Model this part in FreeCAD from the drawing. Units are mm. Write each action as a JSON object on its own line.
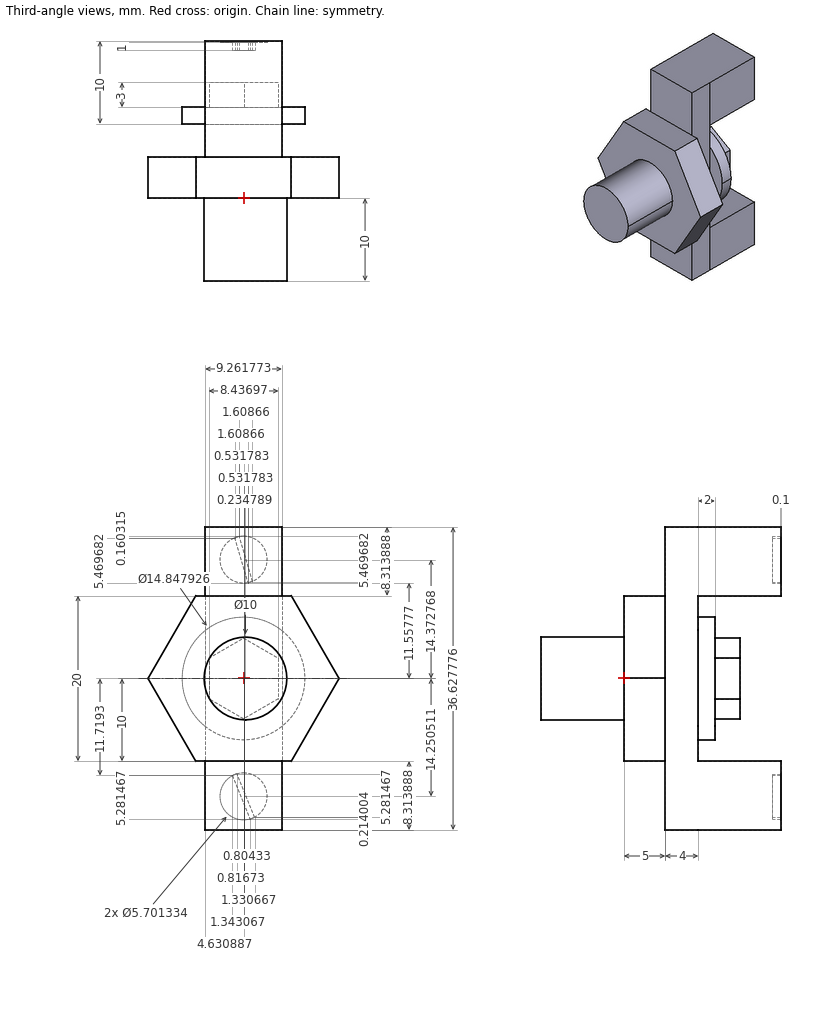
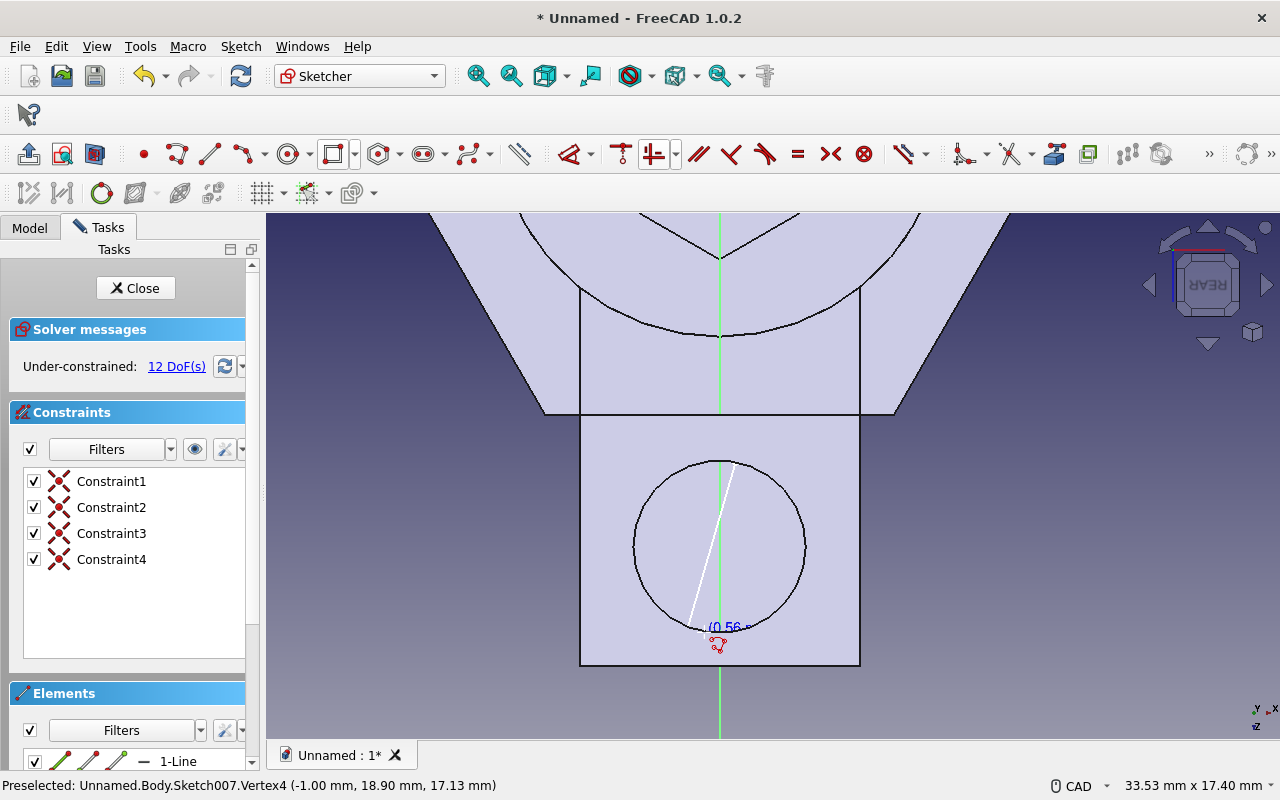
{"action": "left_click", "coordinate": [703, 632]}
{"action": "left_click", "coordinate": [752, 467]}
{"action": "left_click", "coordinate": [735, 463]}
{"action": "key", "text": "Escape"}
{"action": "key", "text": "Escape"}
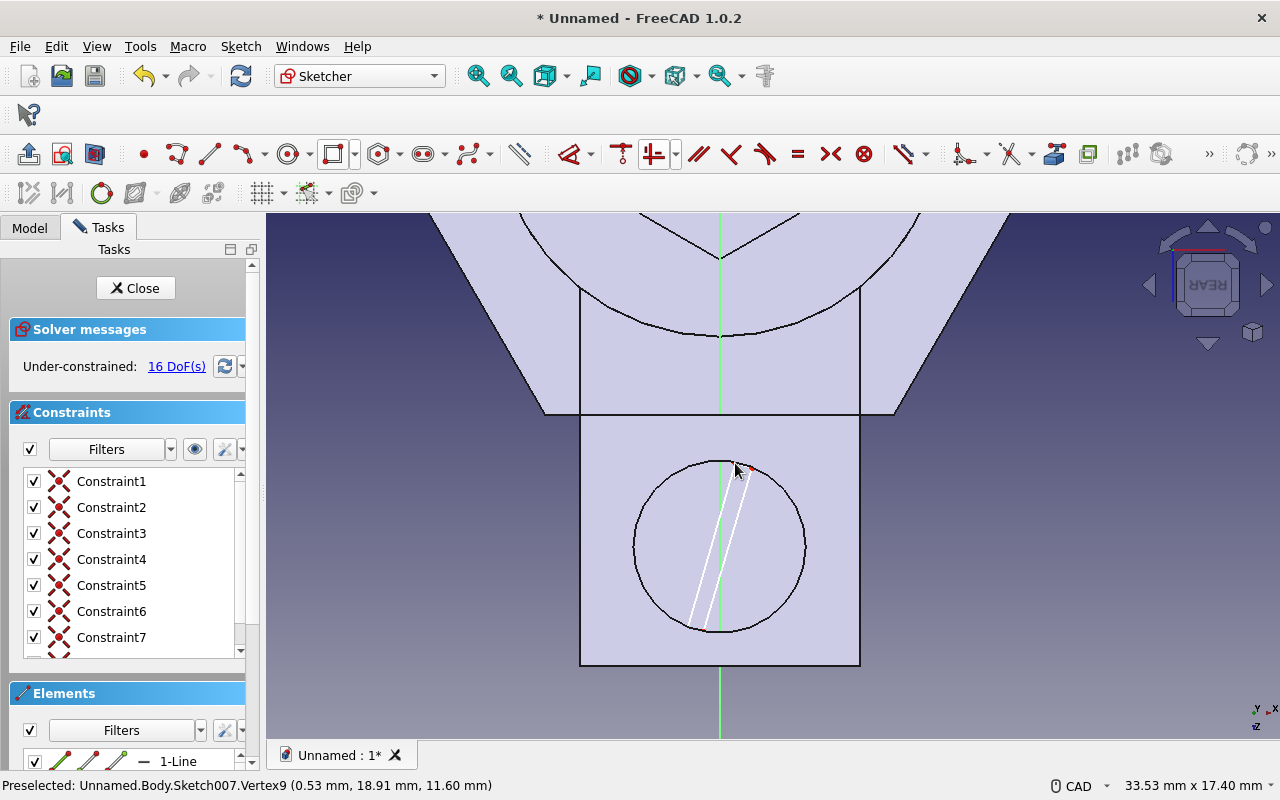
{"action": "left_click", "coordinate": [568, 154]}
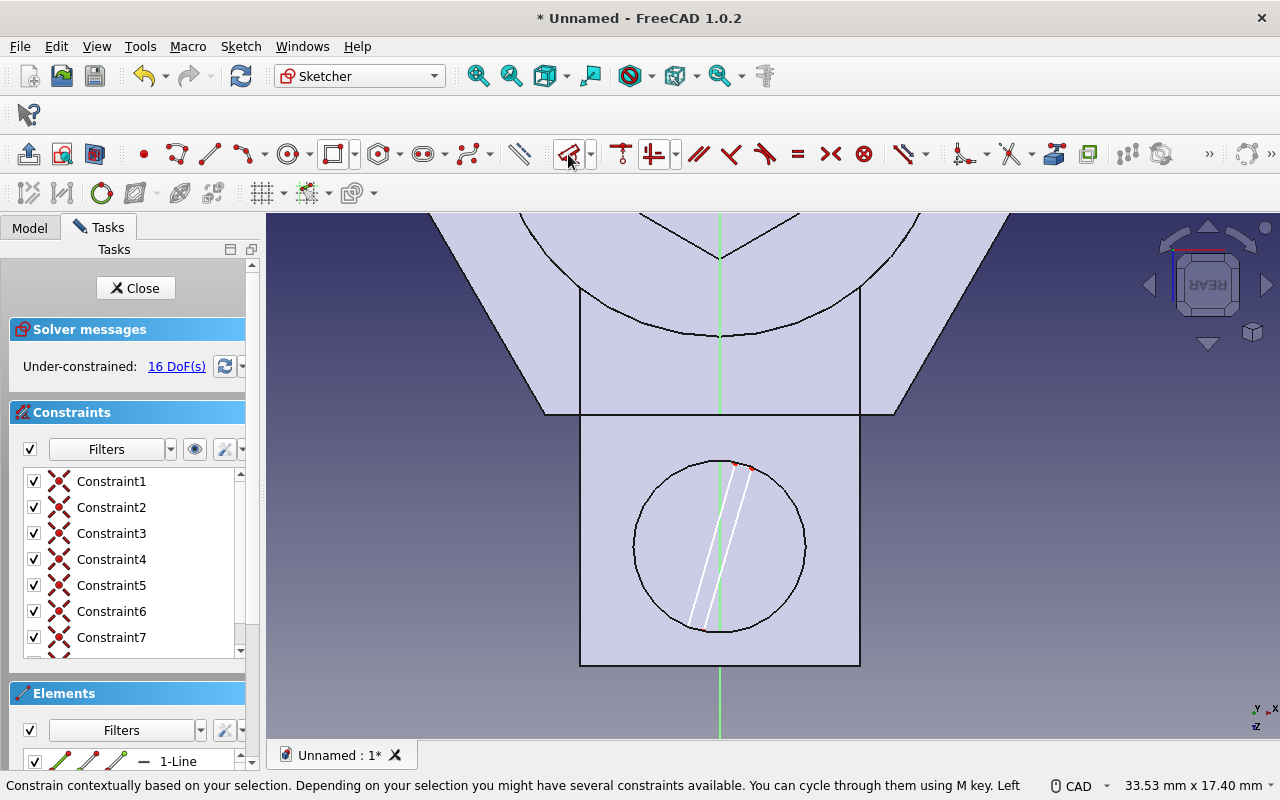
{"action": "scroll", "coordinate": [698, 632], "scroll_direction": "down", "scroll_amount": 6}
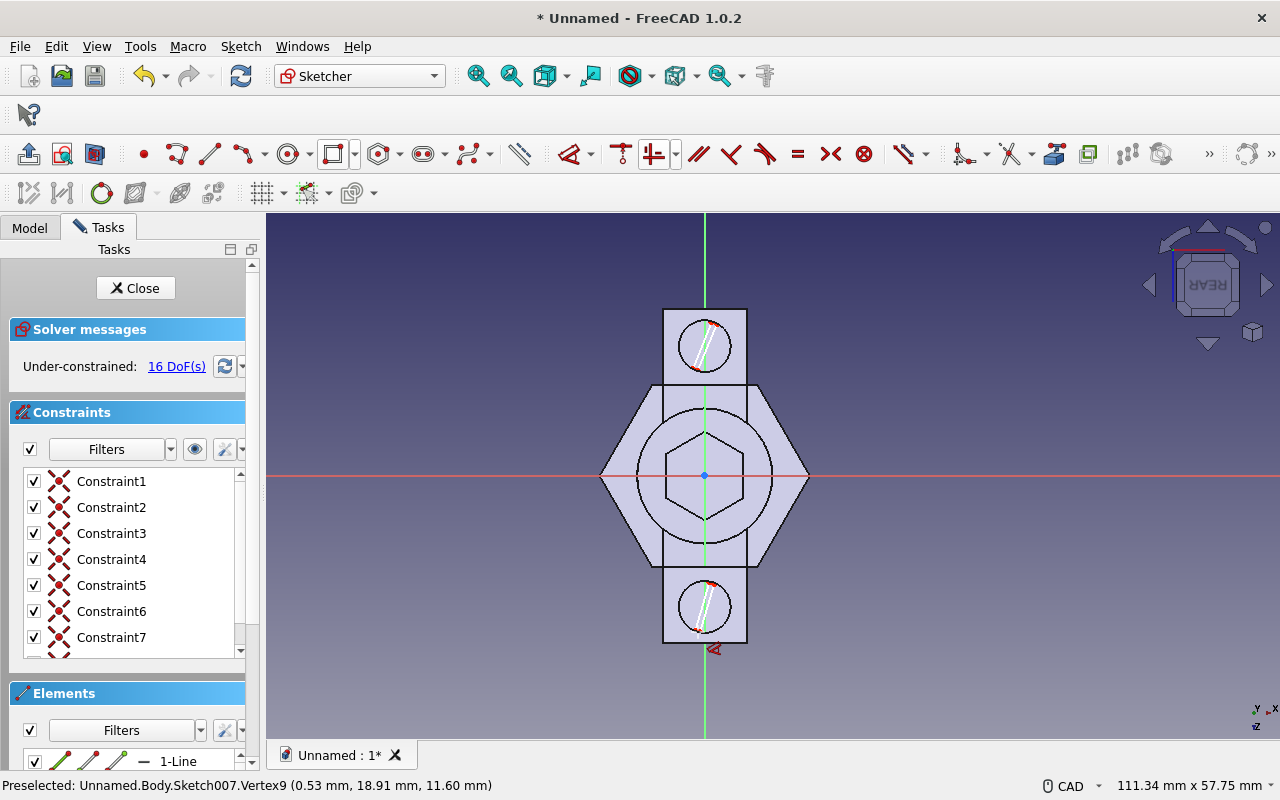
{"action": "scroll", "coordinate": [697, 372], "scroll_direction": "up", "scroll_amount": 9}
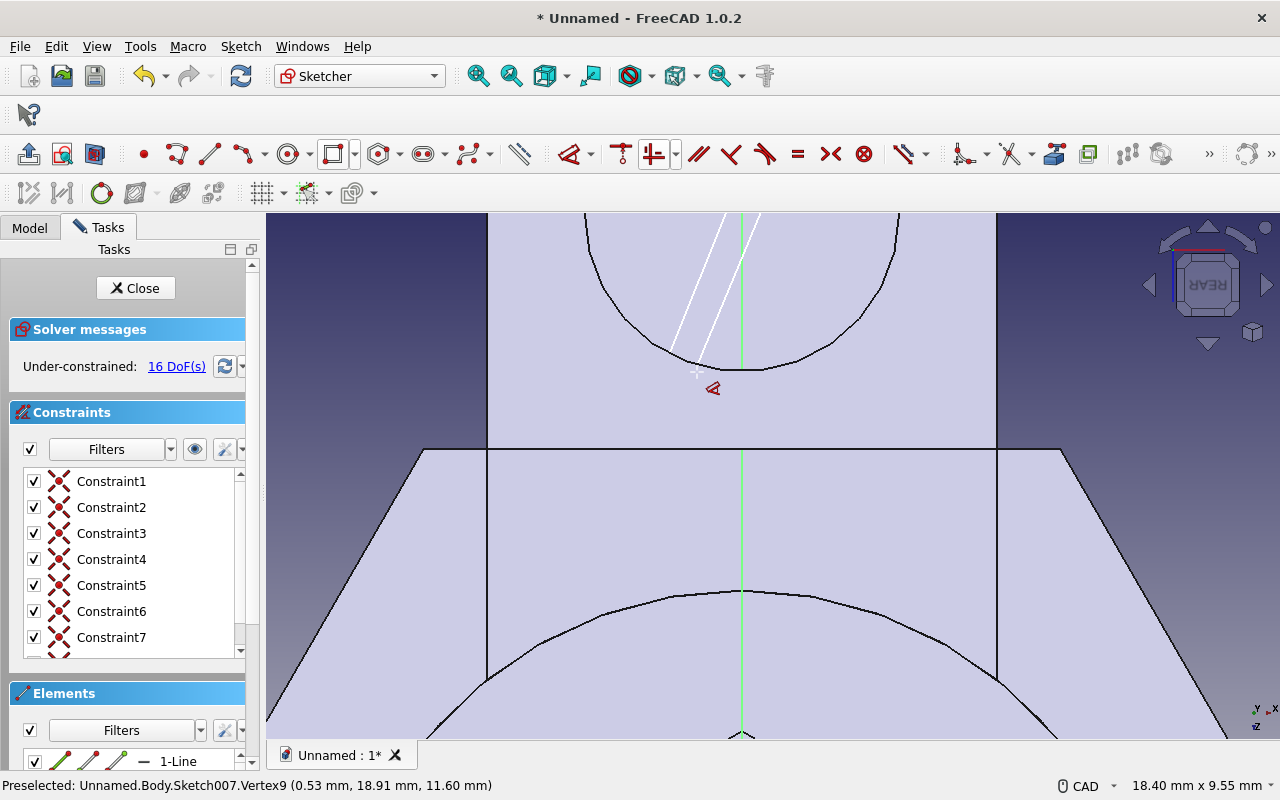
{"action": "left_click", "coordinate": [696, 369]}
{"action": "left_click", "coordinate": [703, 311]}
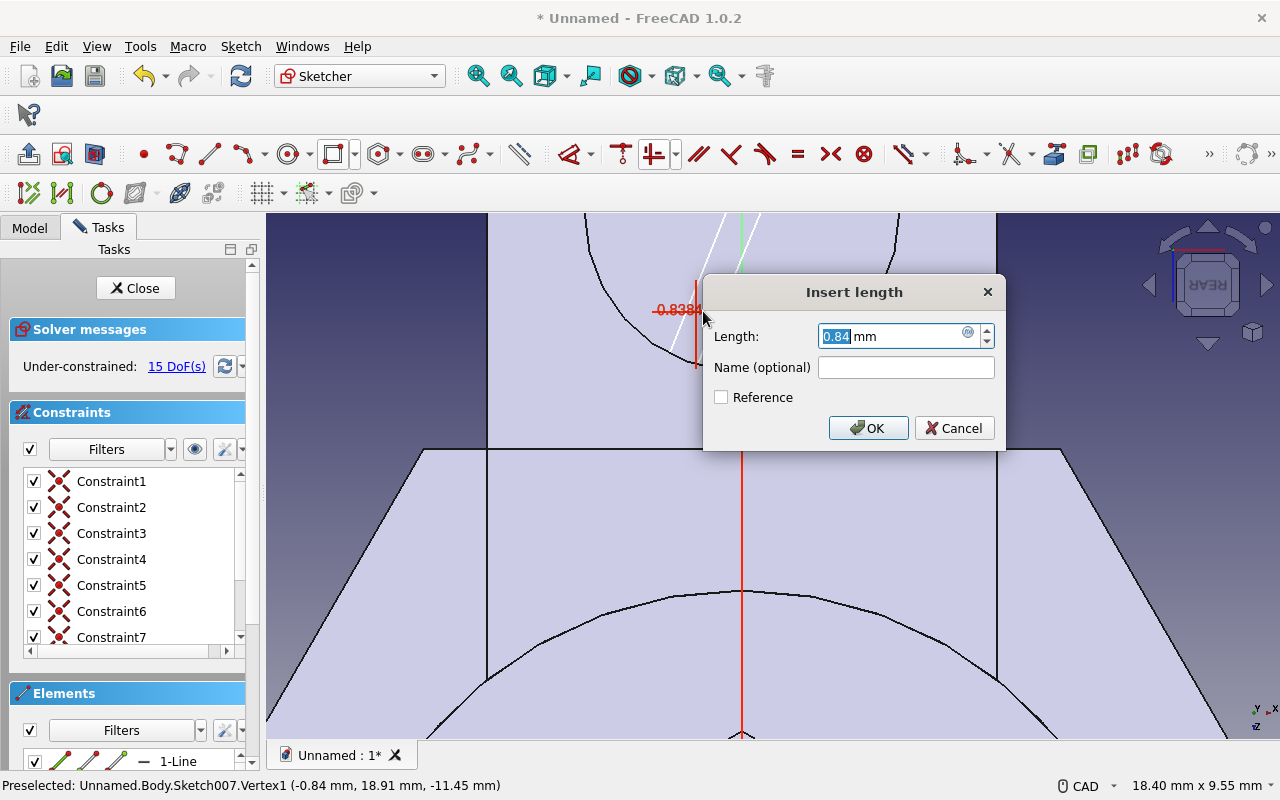
{"action": "type", "text": "0.81673"}
{"action": "key", "text": "Return"}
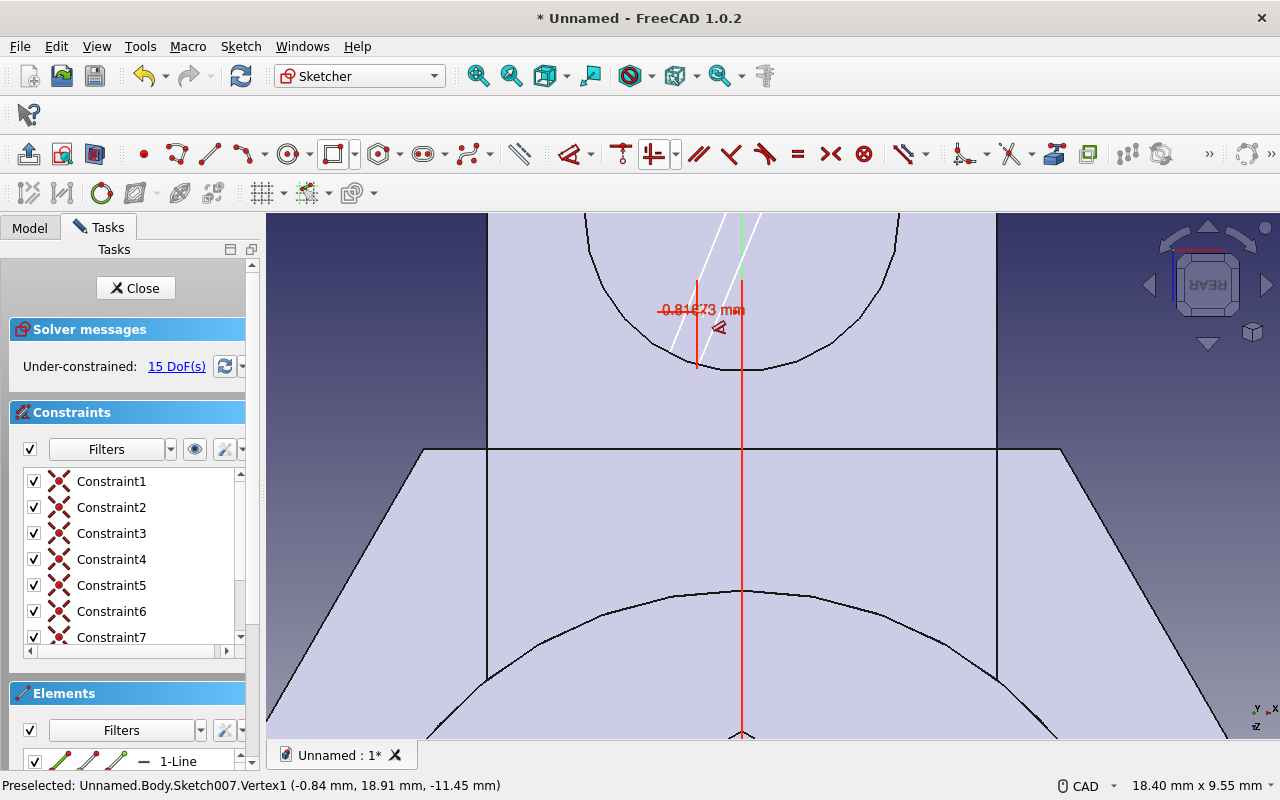
{"action": "scroll", "coordinate": [697, 371], "scroll_direction": "down", "scroll_amount": 9}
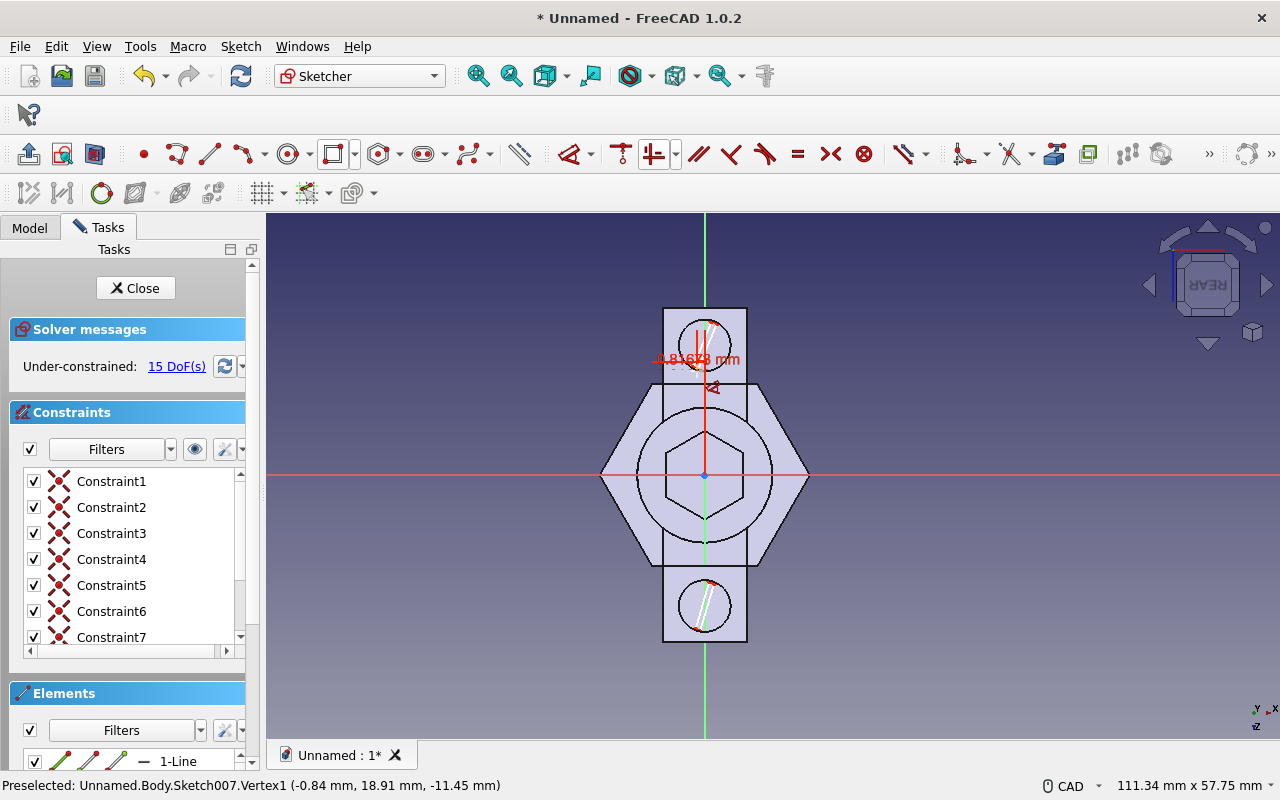
{"action": "scroll", "coordinate": [712, 321], "scroll_direction": "up", "scroll_amount": 9}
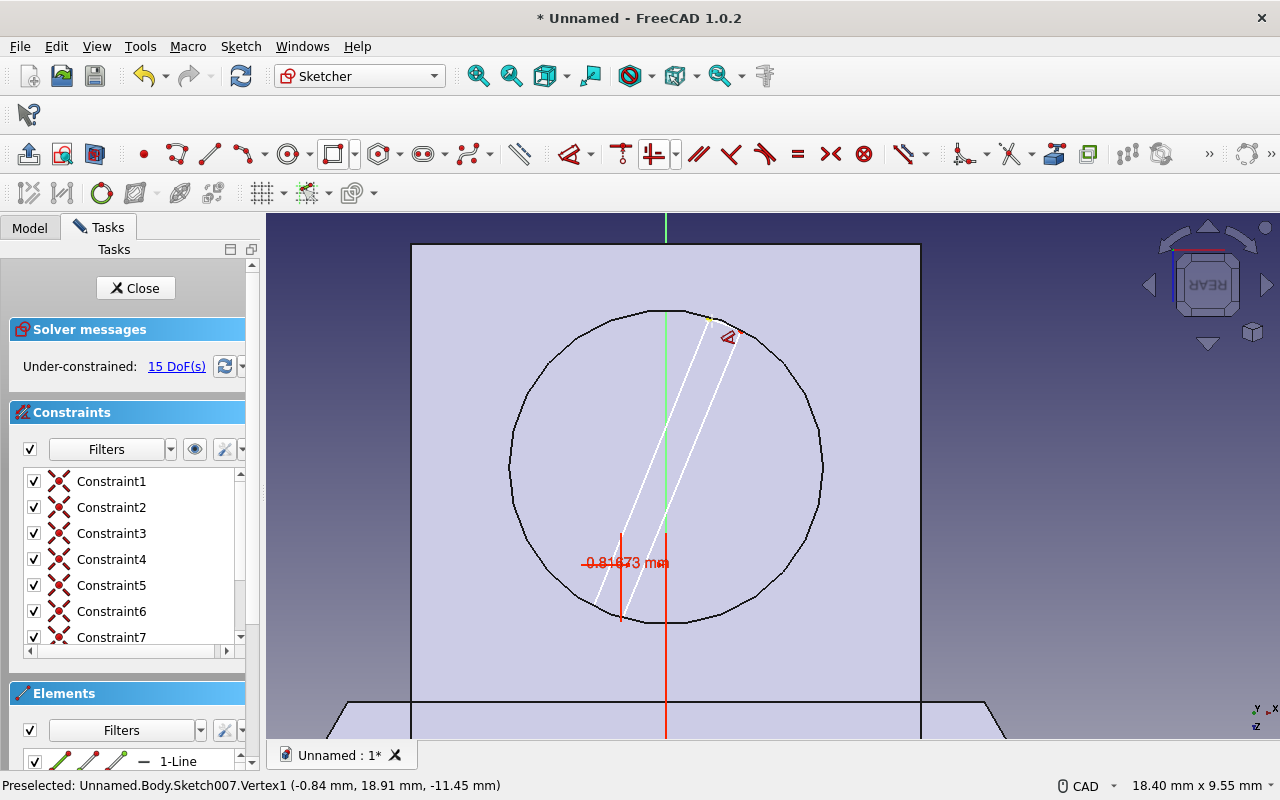
{"action": "left_click", "coordinate": [710, 319]}
{"action": "left_click", "coordinate": [688, 285]}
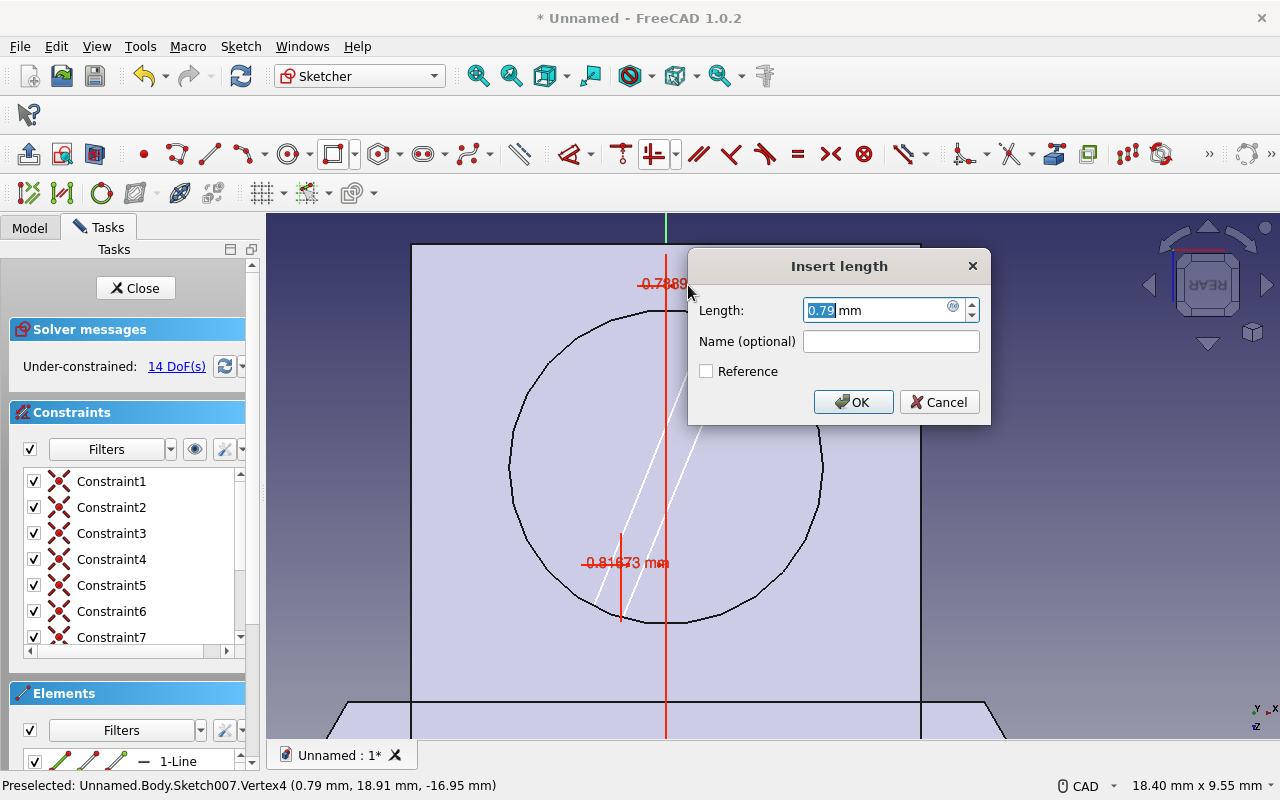
{"action": "type", "text": "0.80433"}
{"action": "key", "text": "Return"}